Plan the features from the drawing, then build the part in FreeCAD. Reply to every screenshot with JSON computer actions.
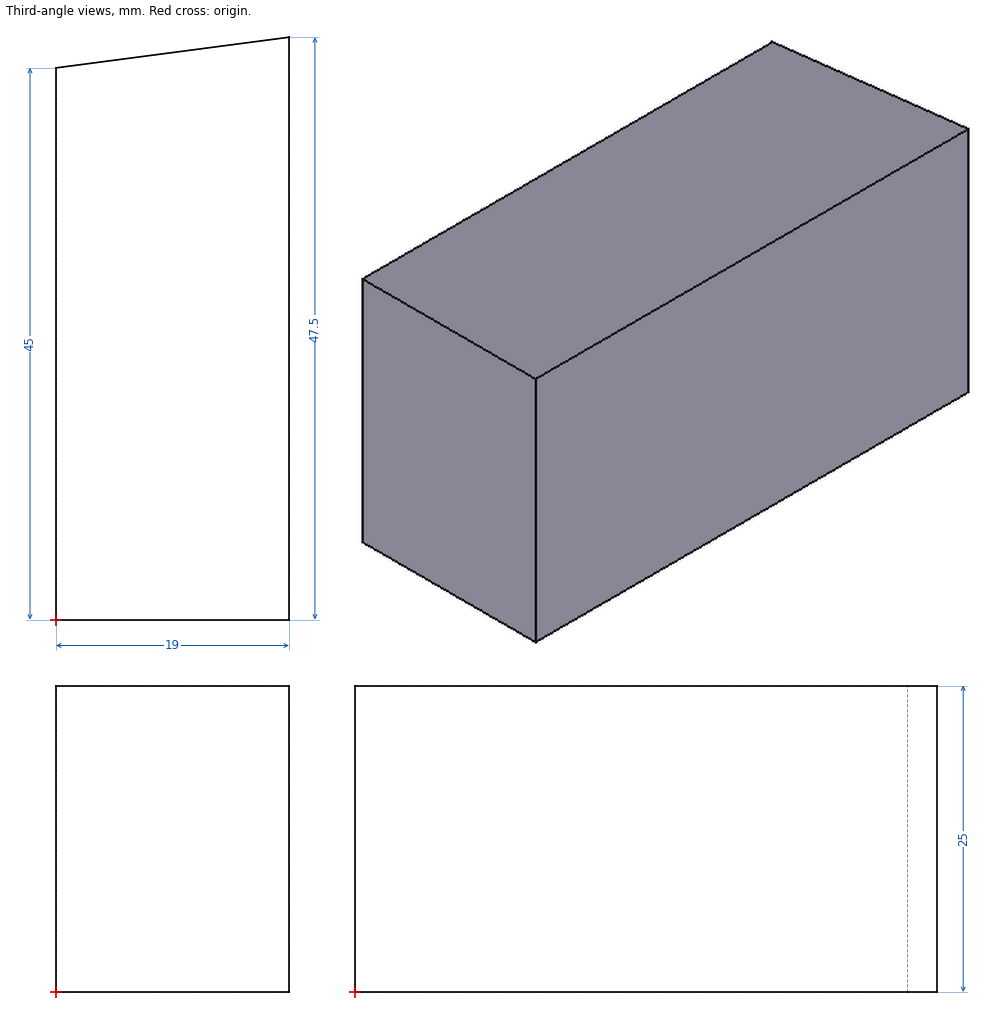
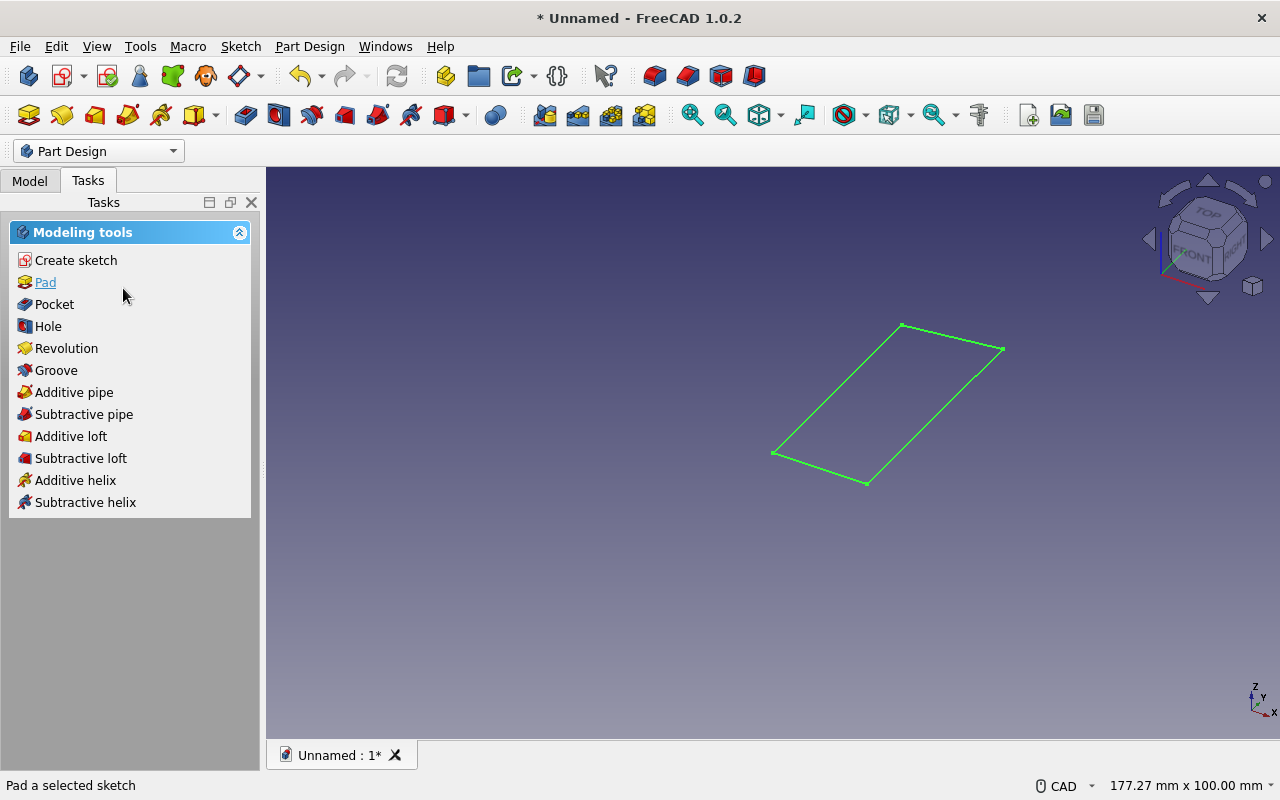
{"action": "left_click", "coordinate": [29, 116]}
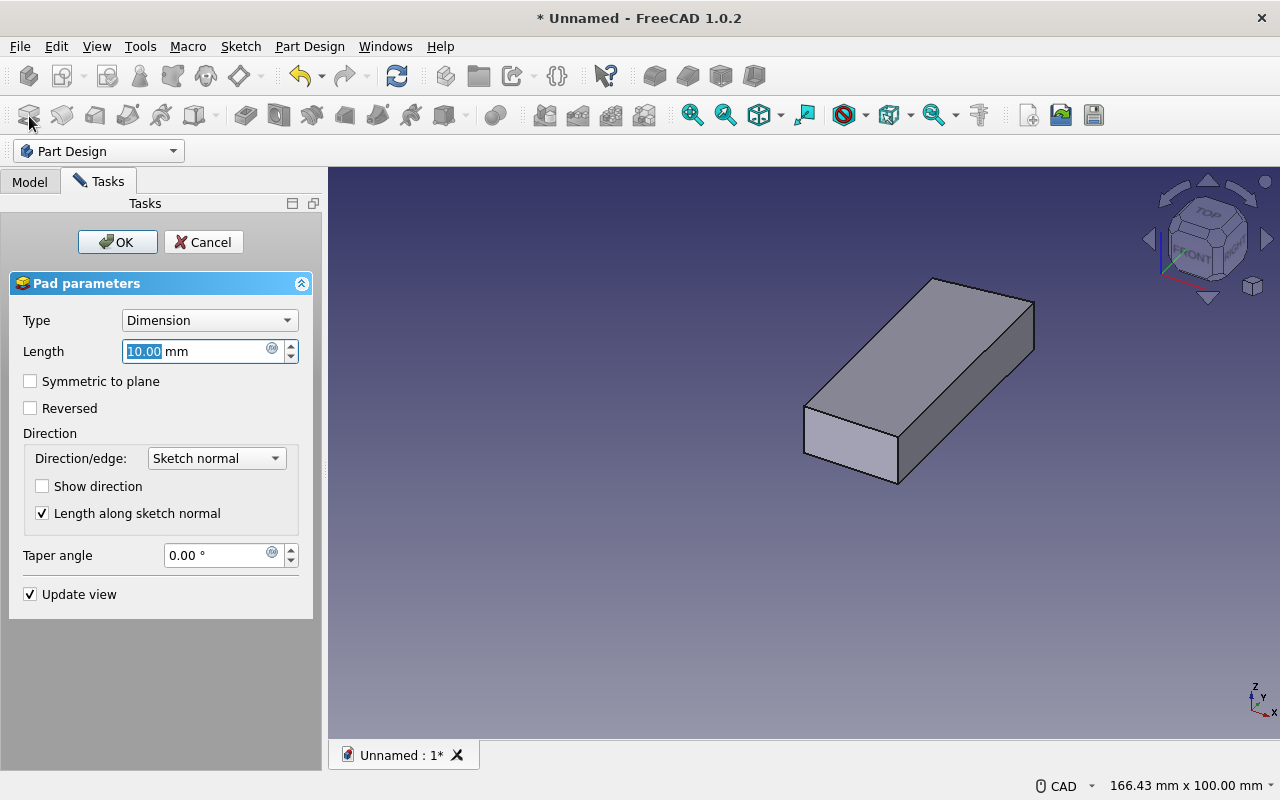
{"action": "type", "text": "25"}
{"action": "key", "text": "Tab"}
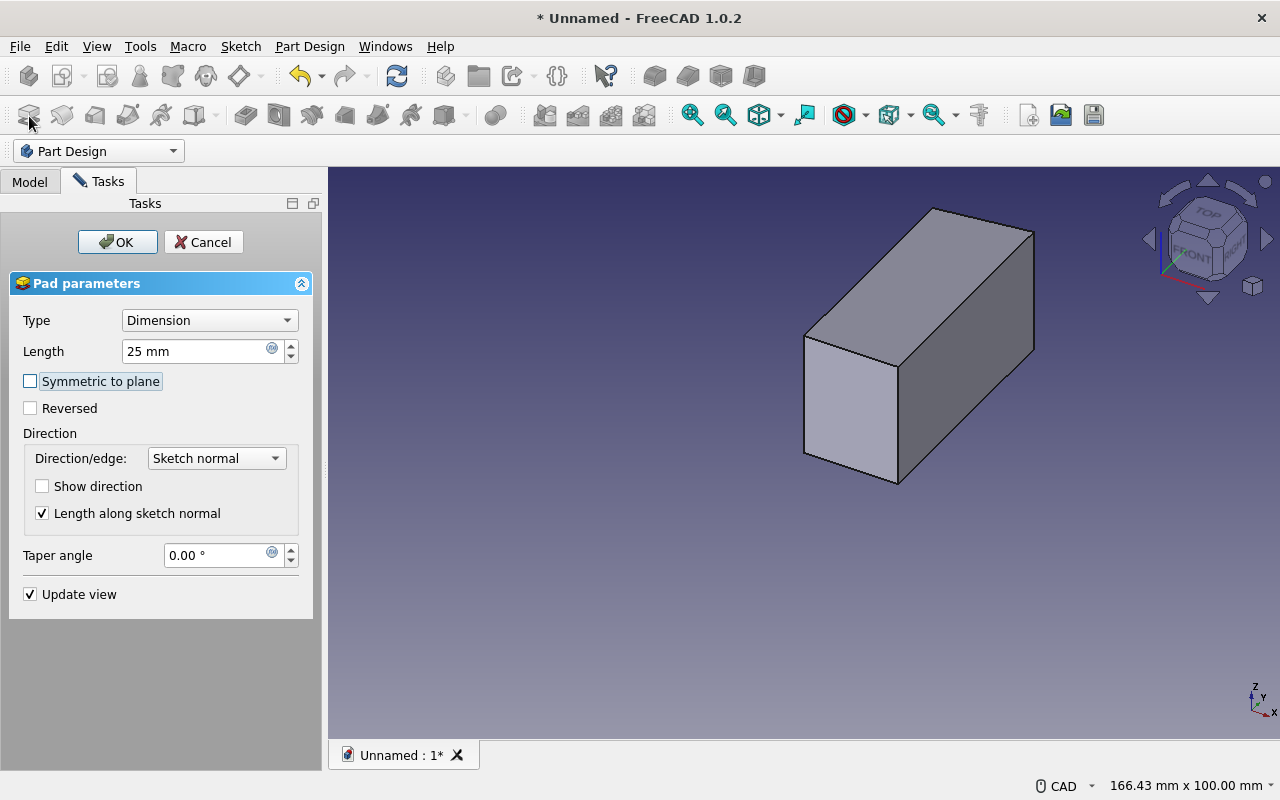
{"action": "left_click", "coordinate": [118, 242]}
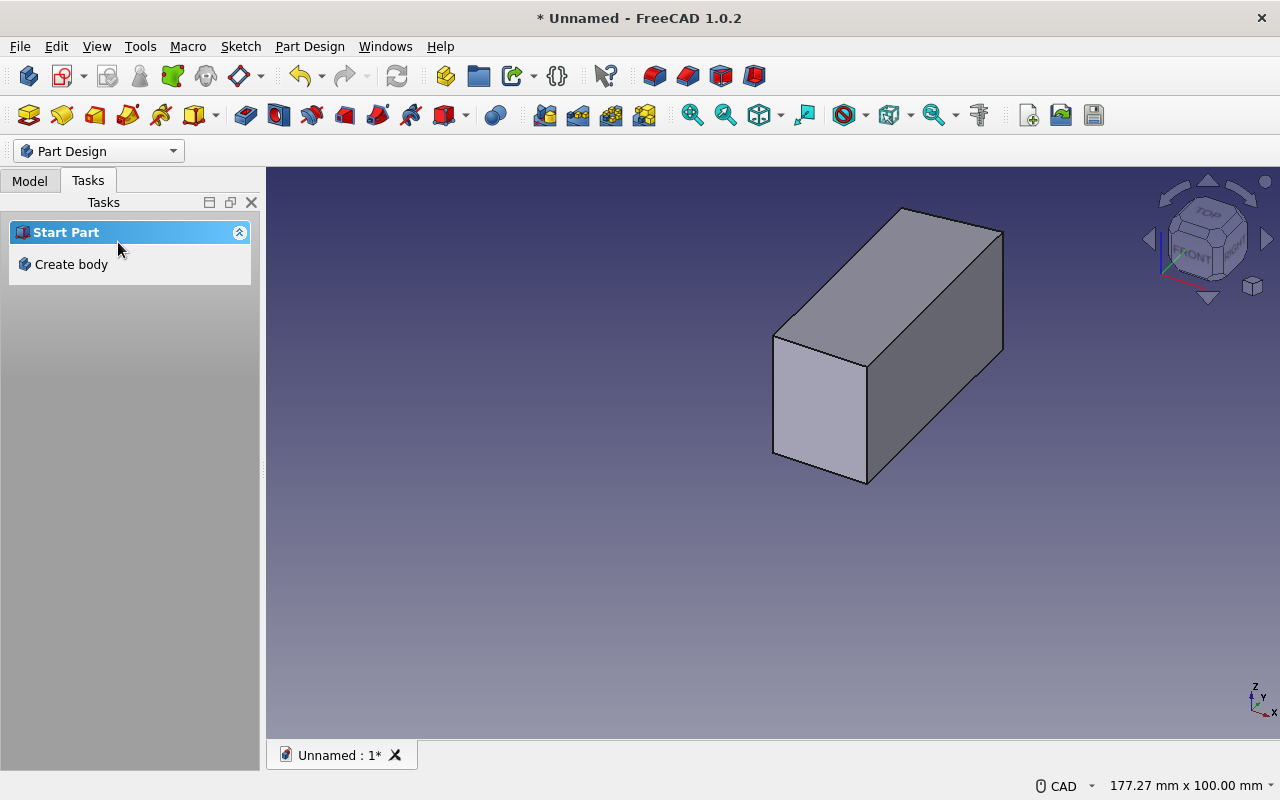
{"action": "key", "text": "0"}